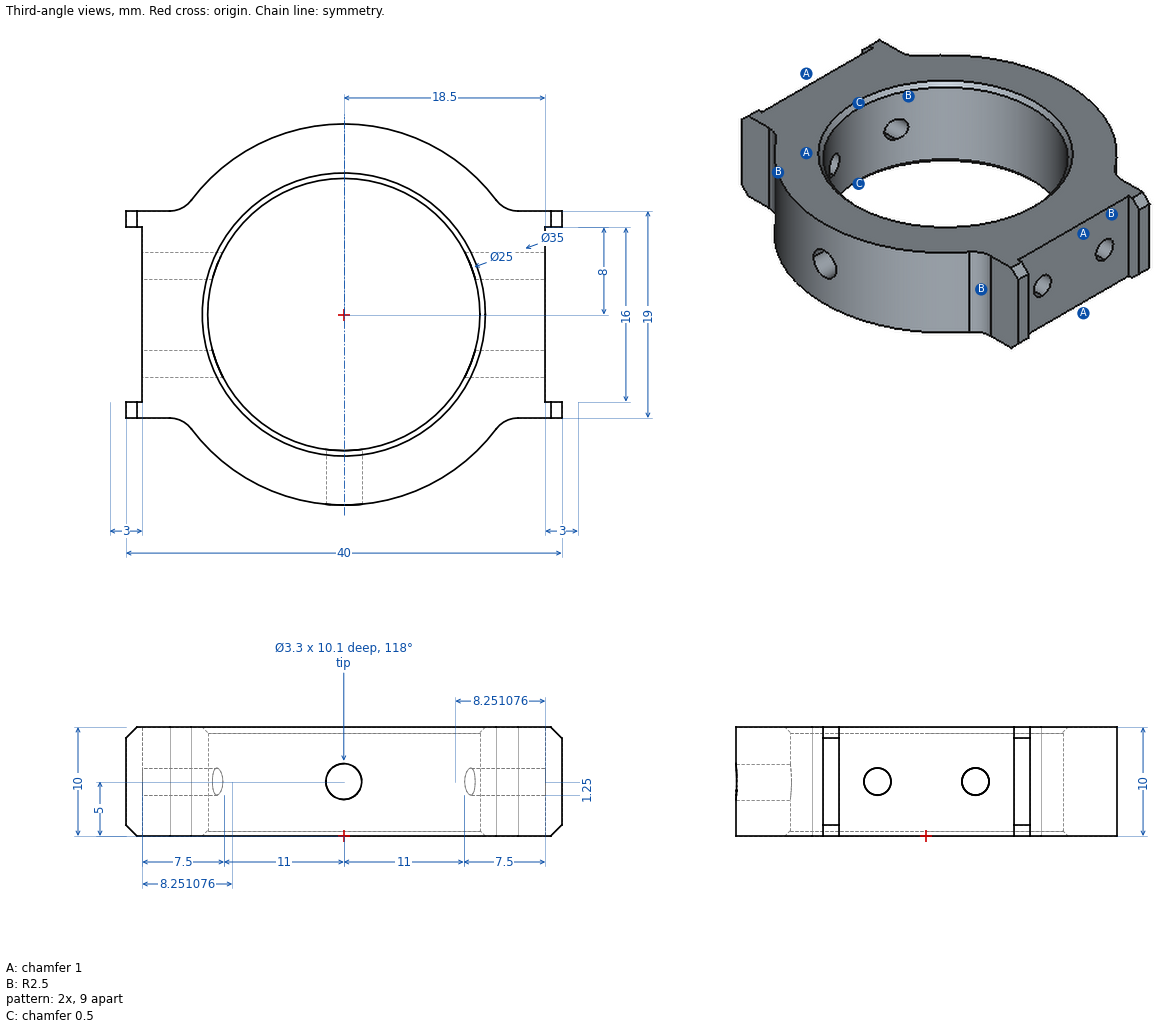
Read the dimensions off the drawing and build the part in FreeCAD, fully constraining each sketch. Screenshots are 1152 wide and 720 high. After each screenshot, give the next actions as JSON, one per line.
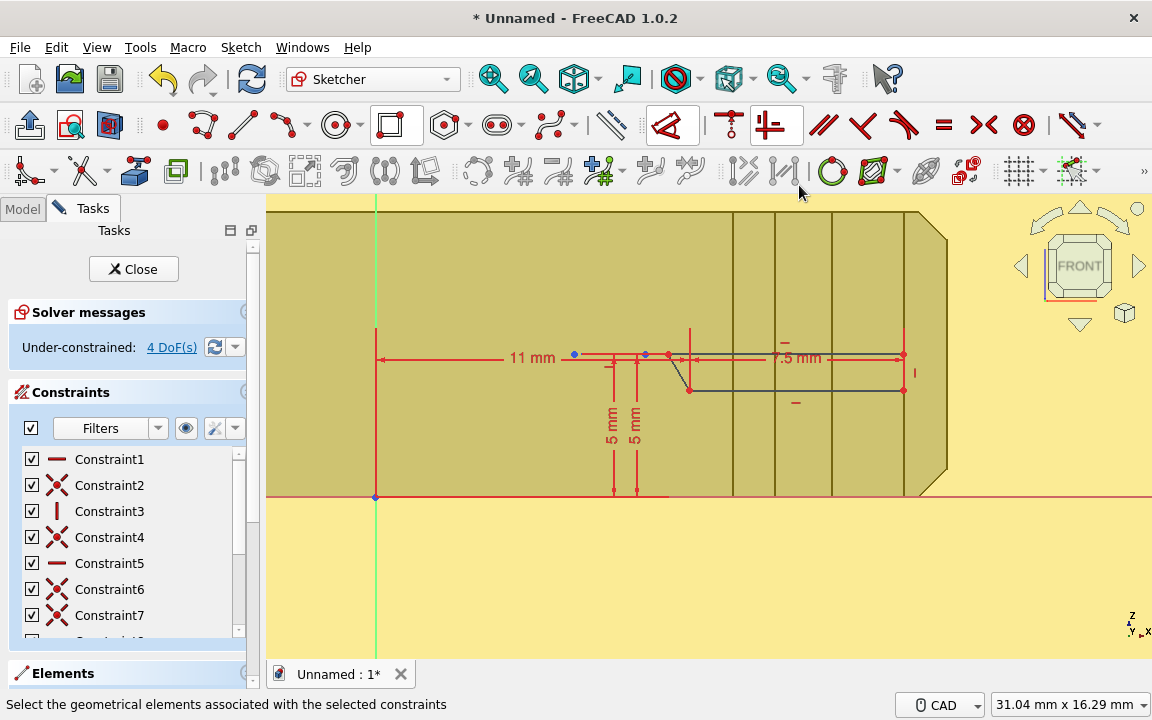
{"action": "scroll", "coordinate": [904, 365], "scroll_direction": "up", "scroll_amount": 2}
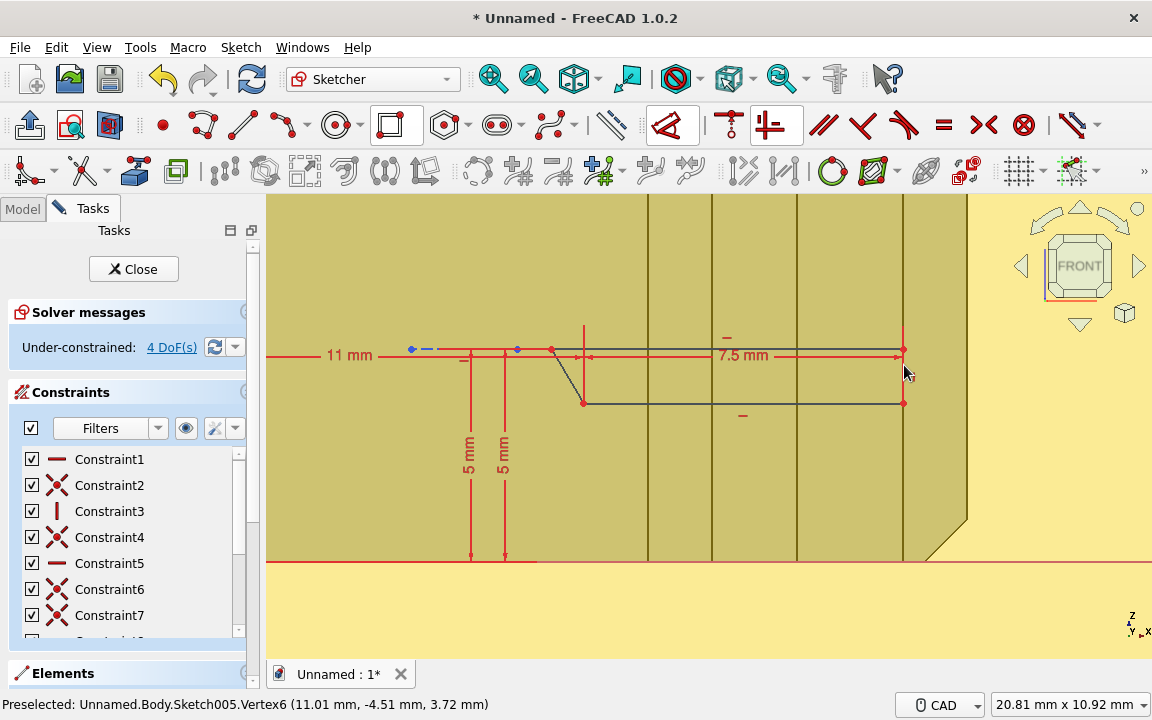
{"action": "left_click", "coordinate": [903, 365]}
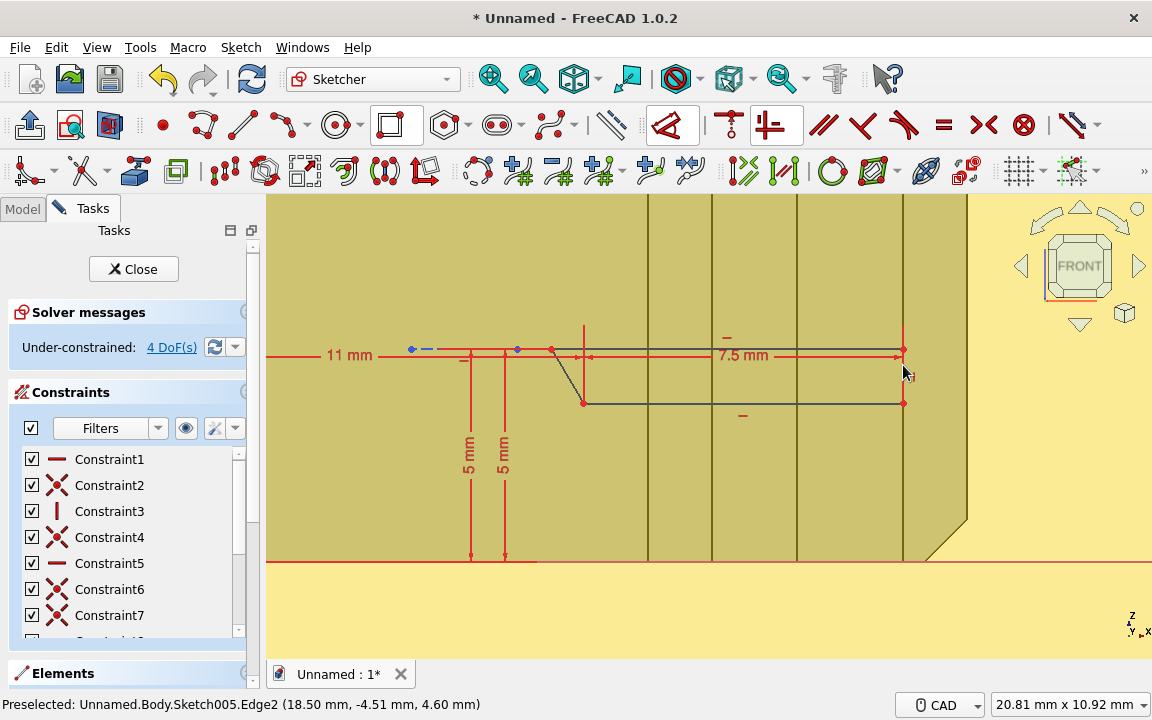
{"action": "left_click", "coordinate": [694, 126]}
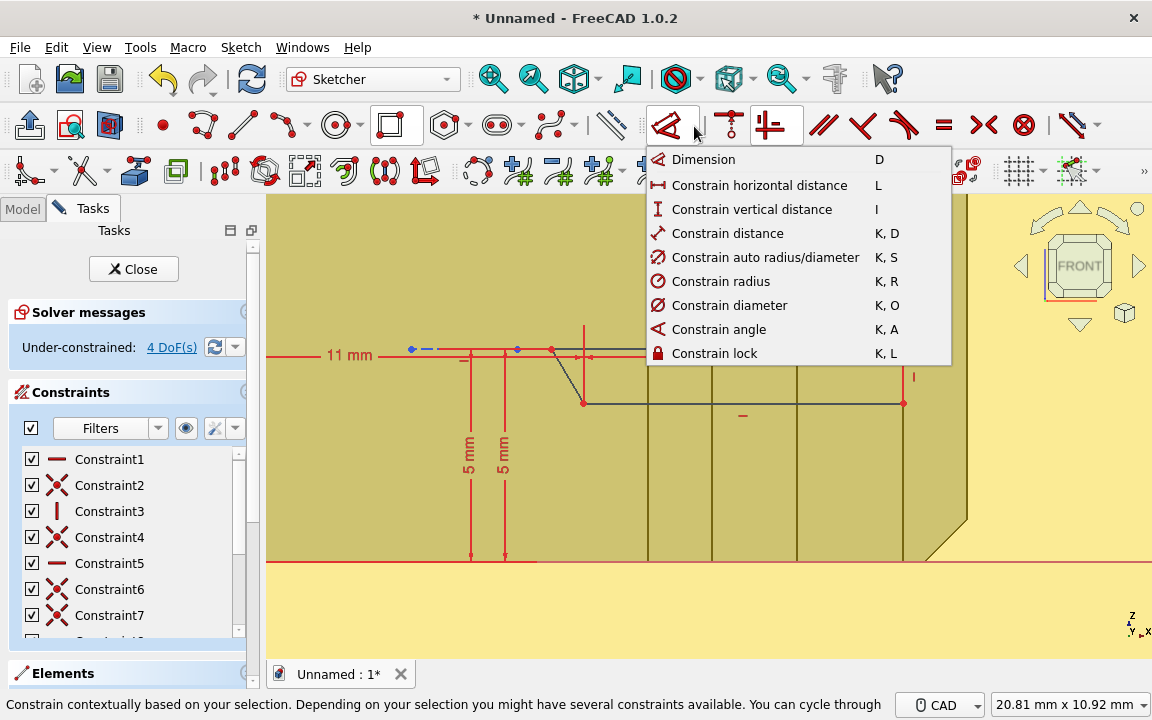
{"action": "left_click", "coordinate": [799, 209]}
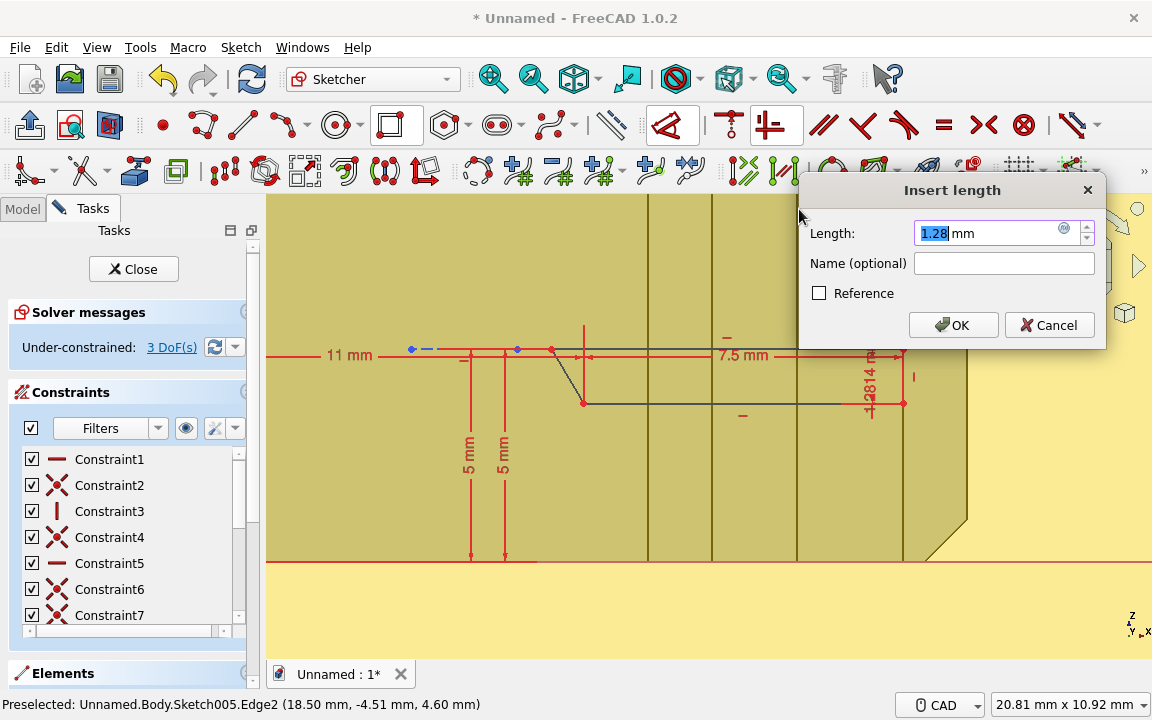
{"action": "type", "text": "1.25"}
{"action": "key", "text": "Return"}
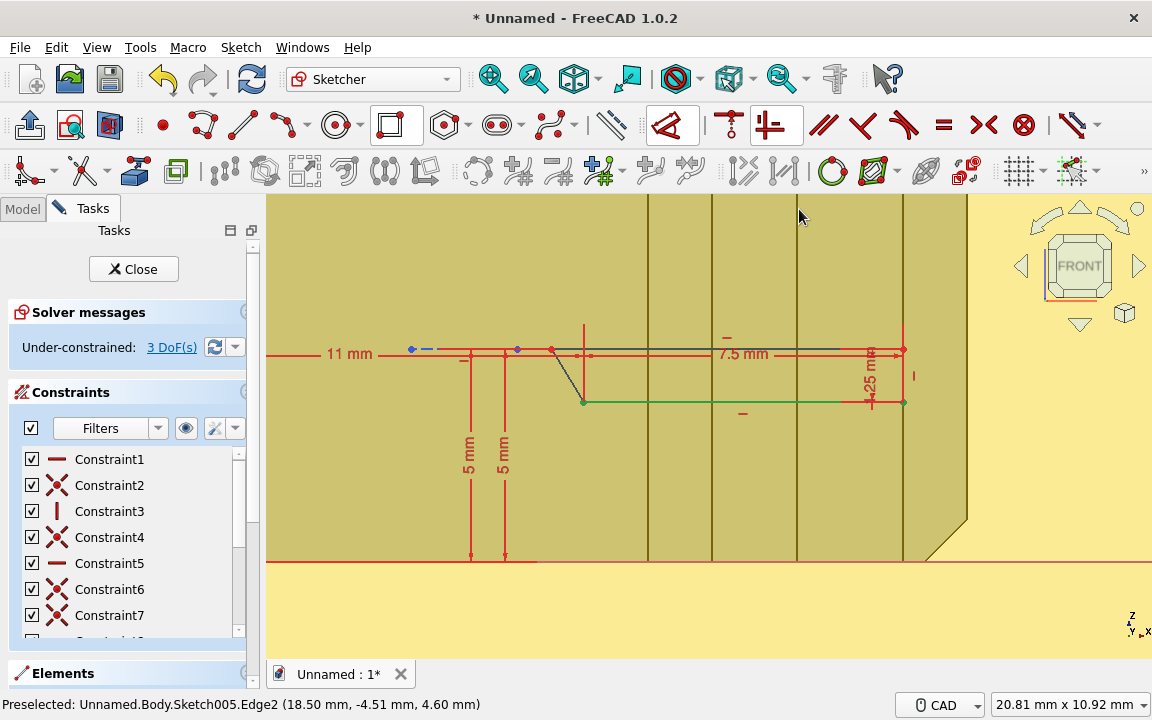
{"action": "left_click", "coordinate": [657, 349]}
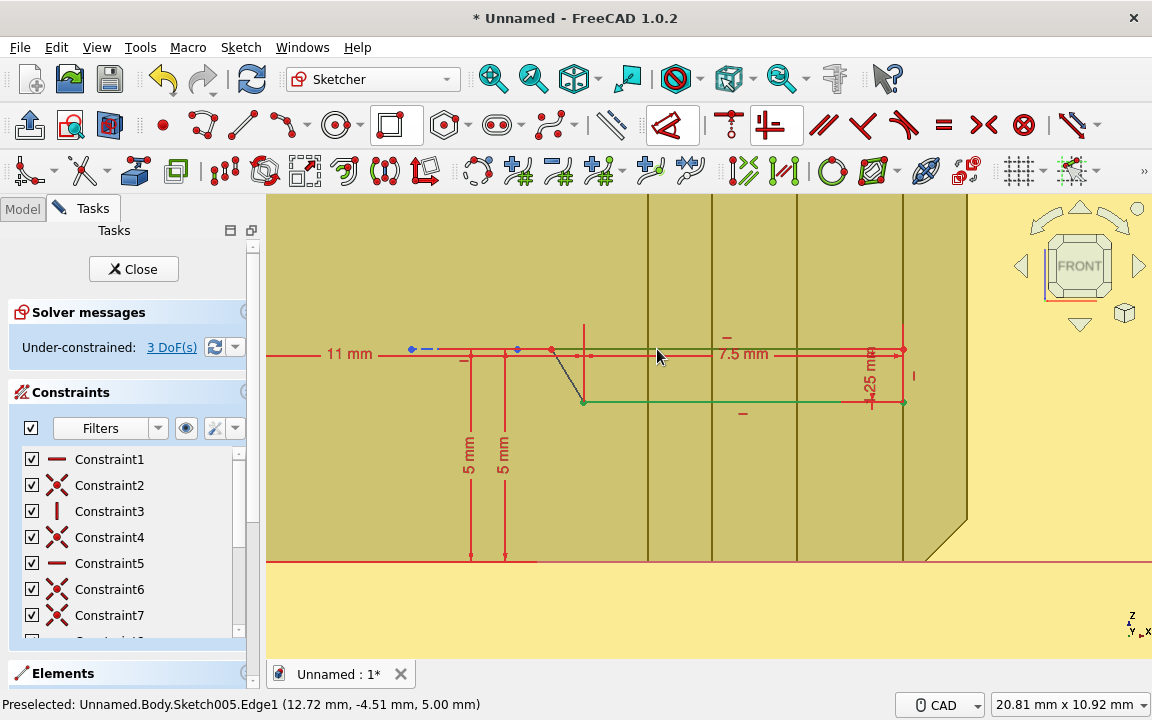
{"action": "key", "text": "l"}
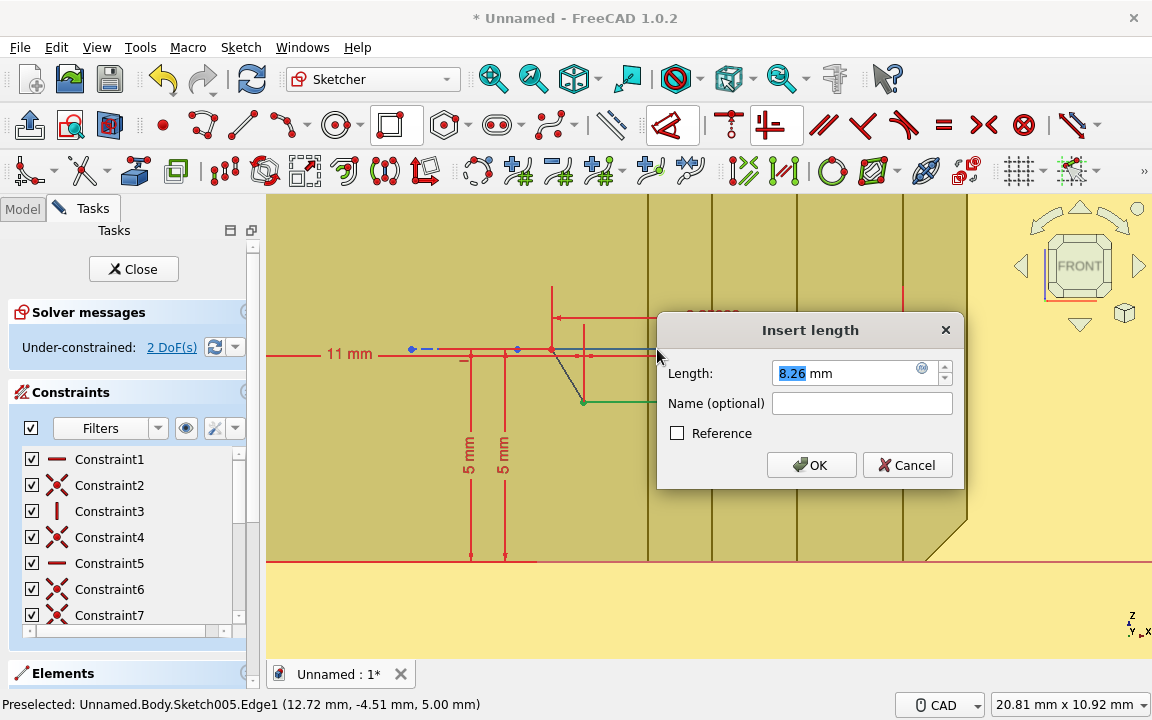
{"action": "type", "text": "8.251076"}
{"action": "key", "text": "Return"}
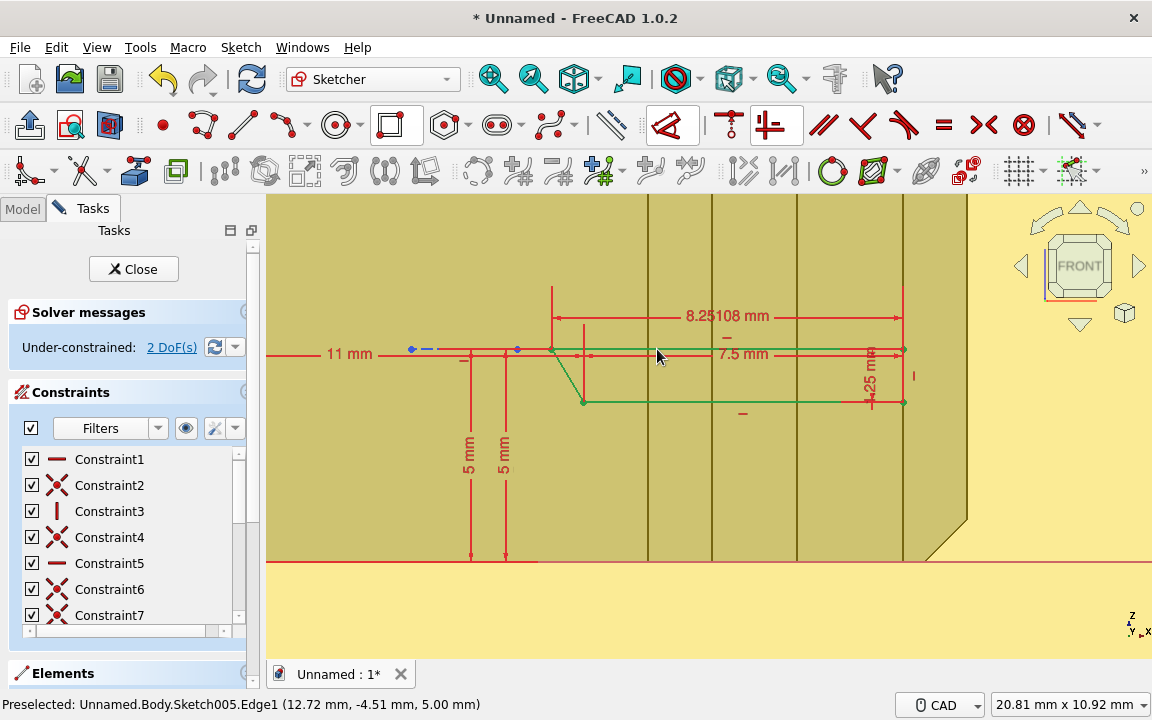
{"action": "left_click", "coordinate": [134, 269]}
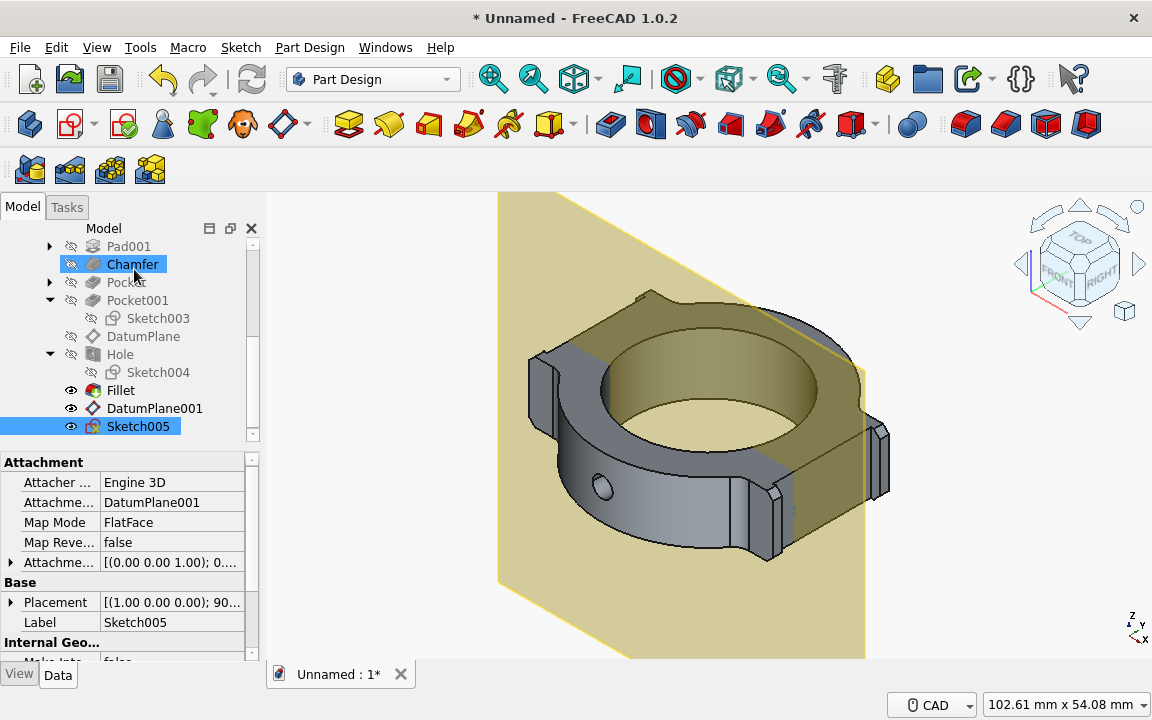
{"action": "left_click", "coordinate": [692, 124]}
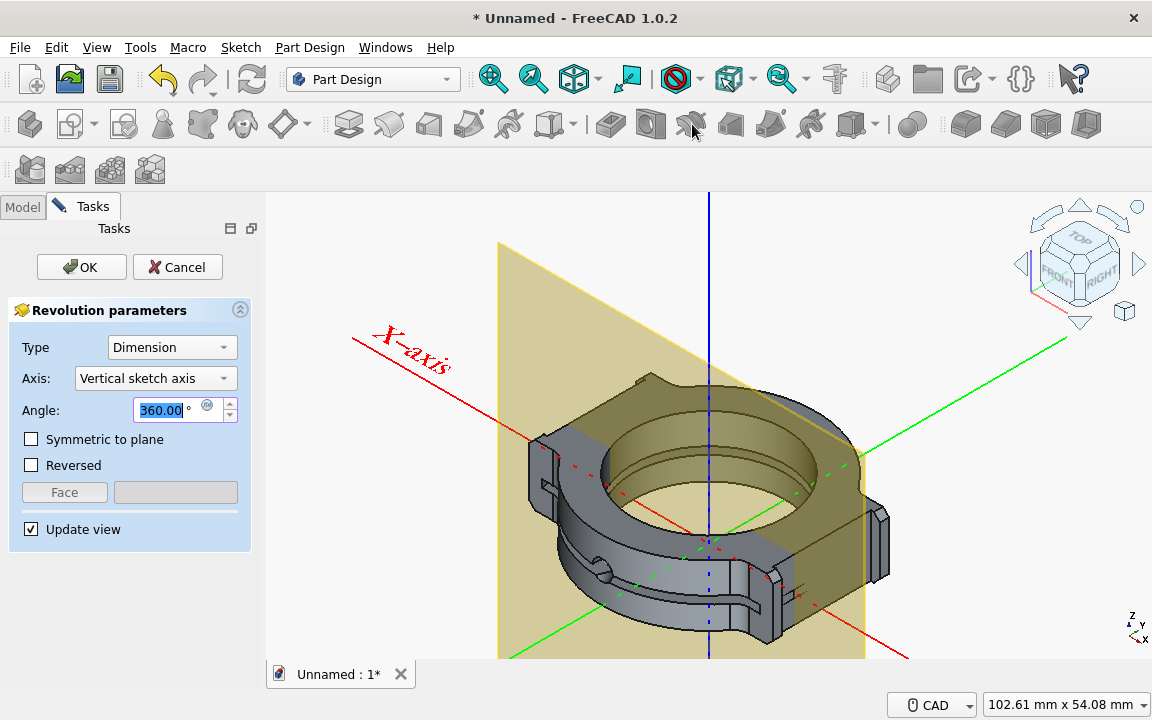
{"action": "left_click", "coordinate": [156, 378]}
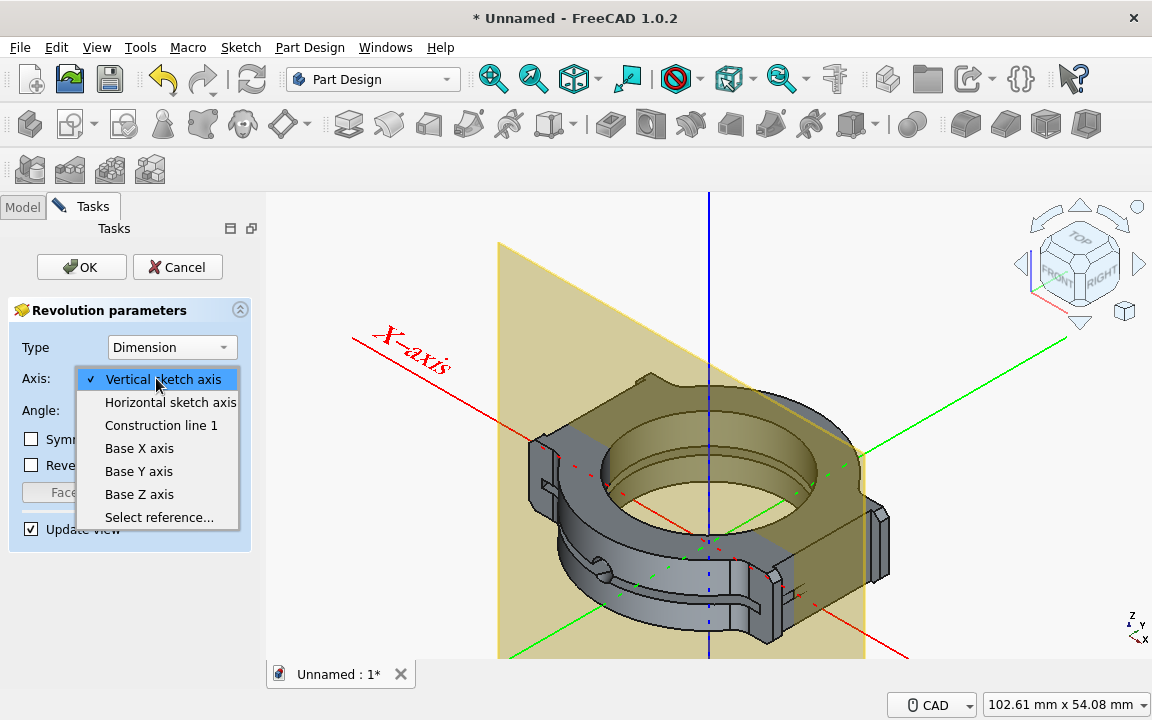
{"action": "left_click", "coordinate": [156, 426]}